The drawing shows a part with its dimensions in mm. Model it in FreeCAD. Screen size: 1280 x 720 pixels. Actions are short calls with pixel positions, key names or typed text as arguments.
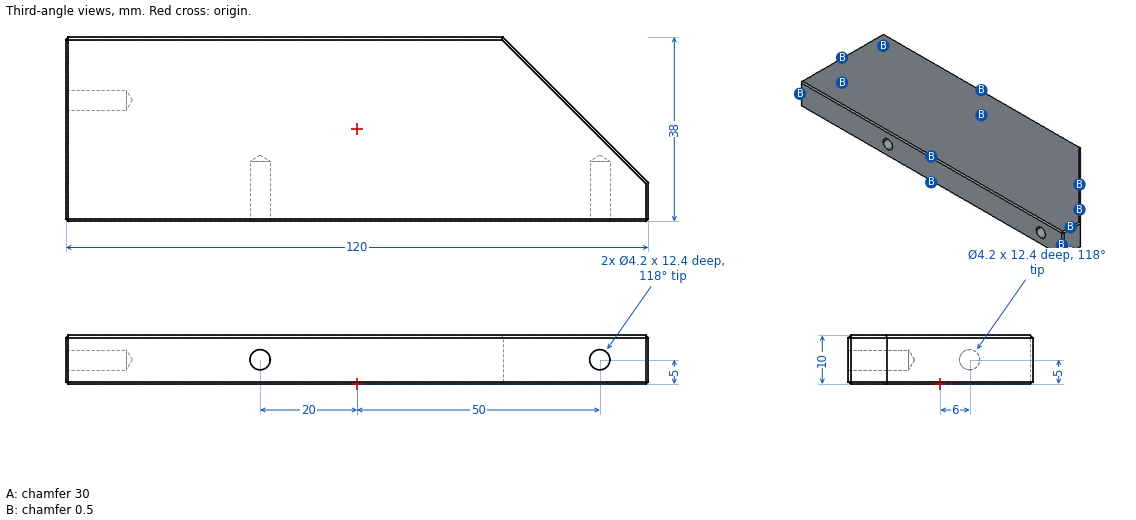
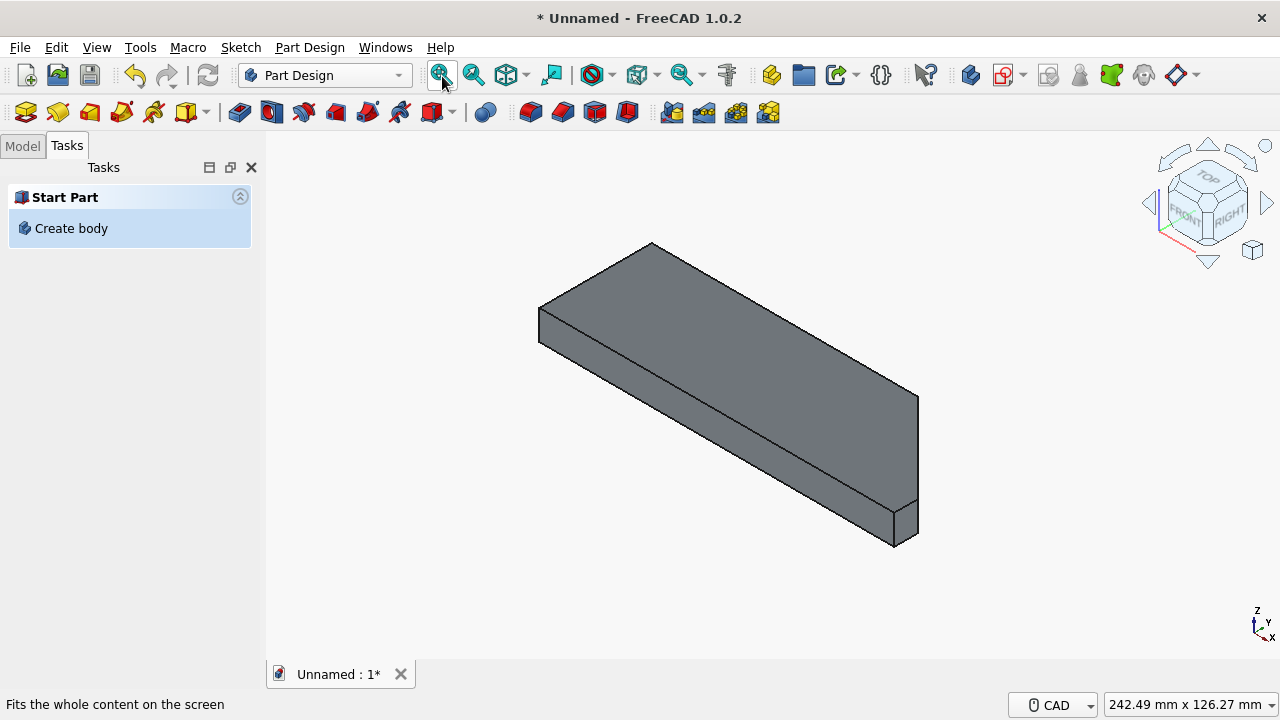
click(869, 514)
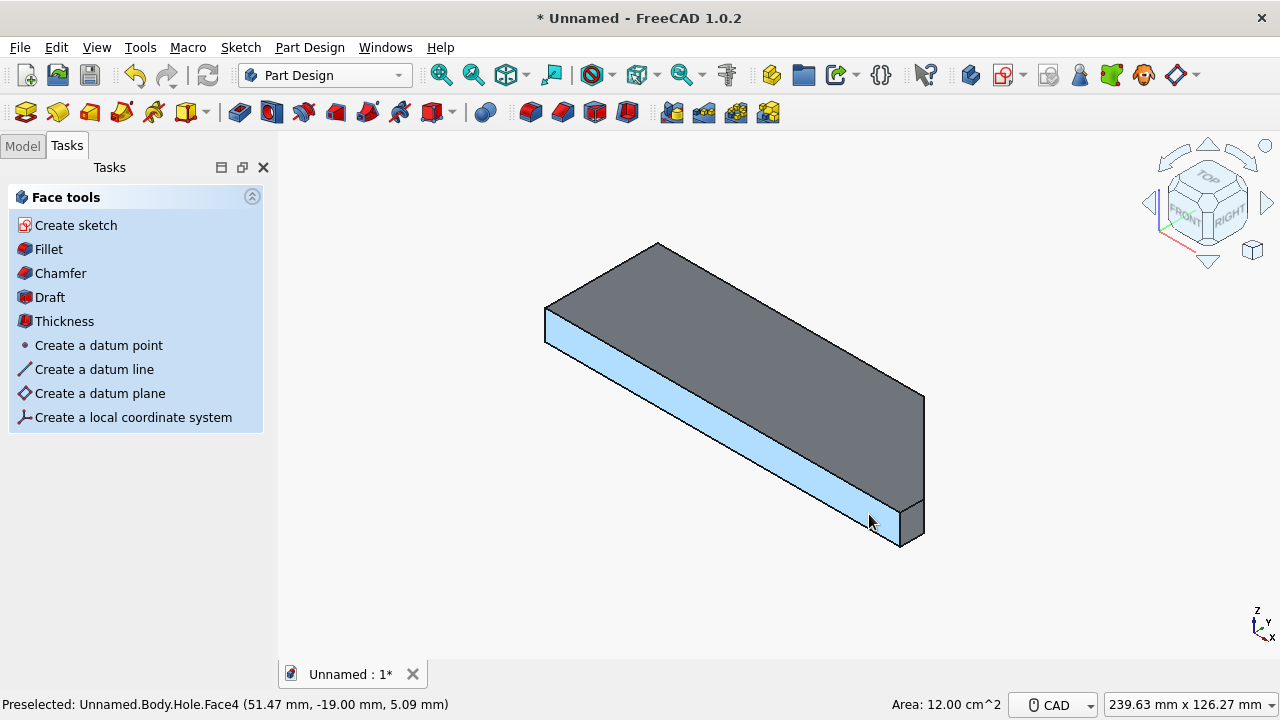
click(1004, 76)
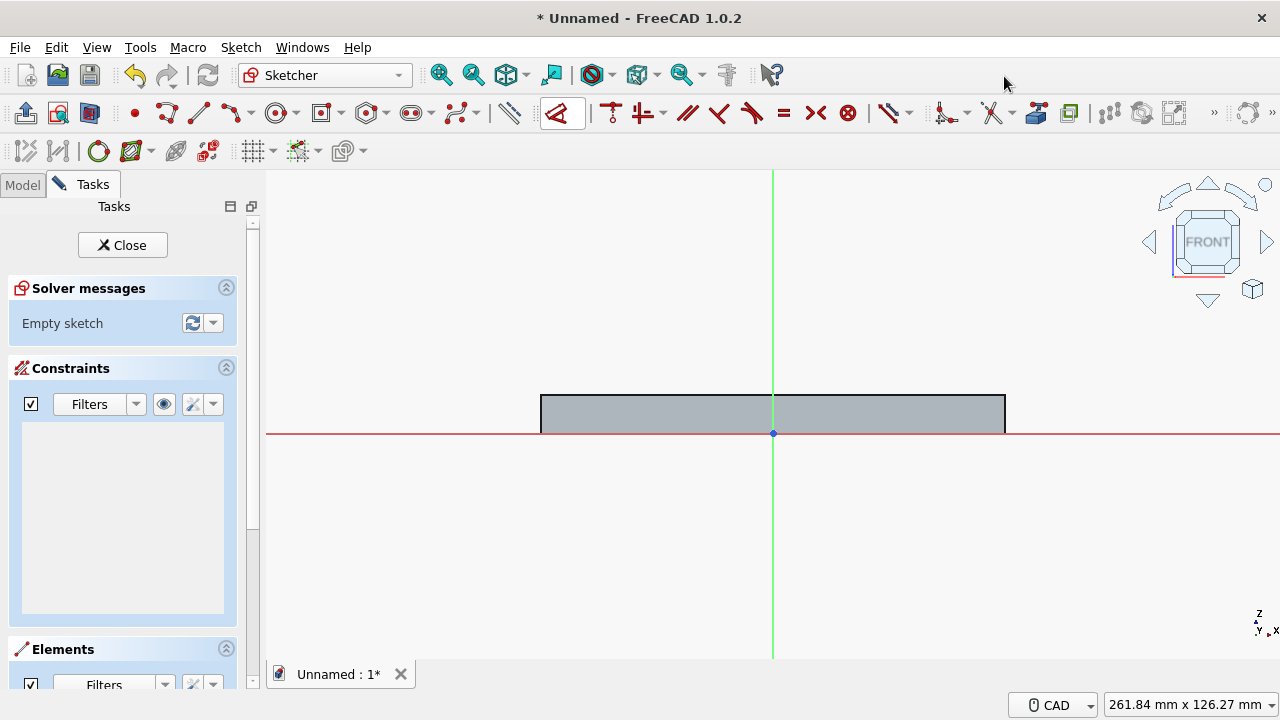
scroll(934, 425, up, 4)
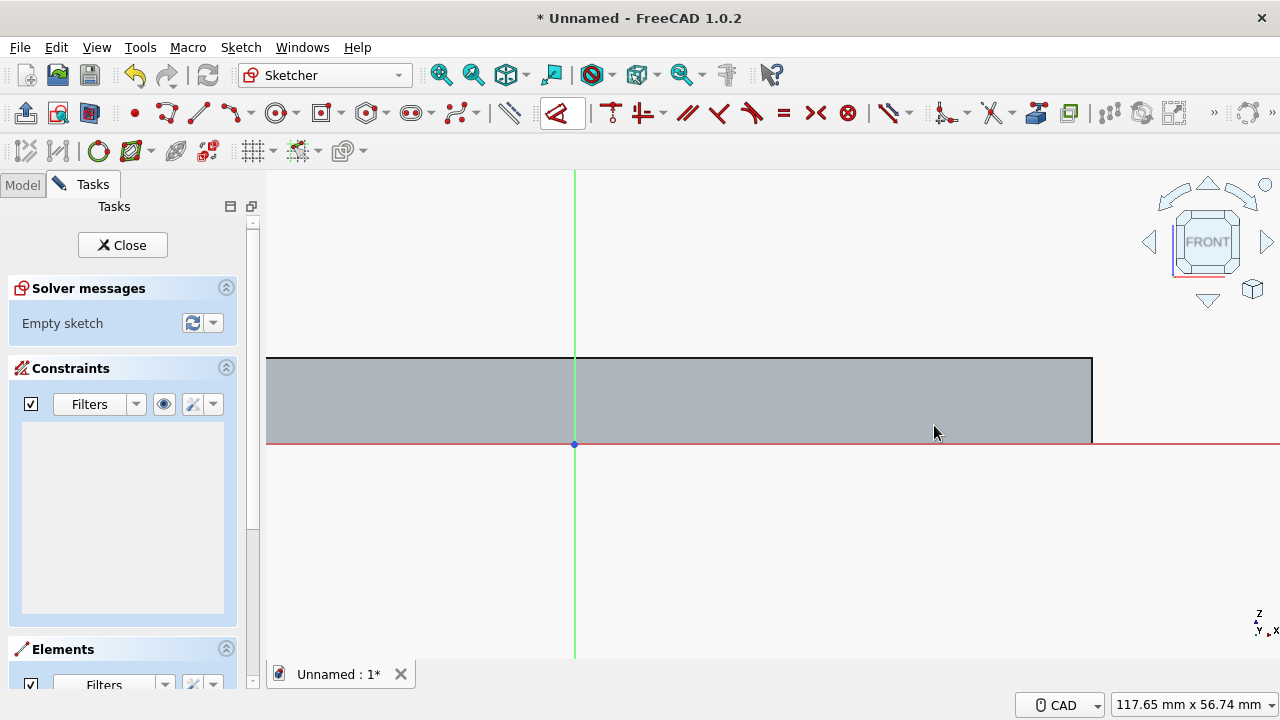
click(276, 114)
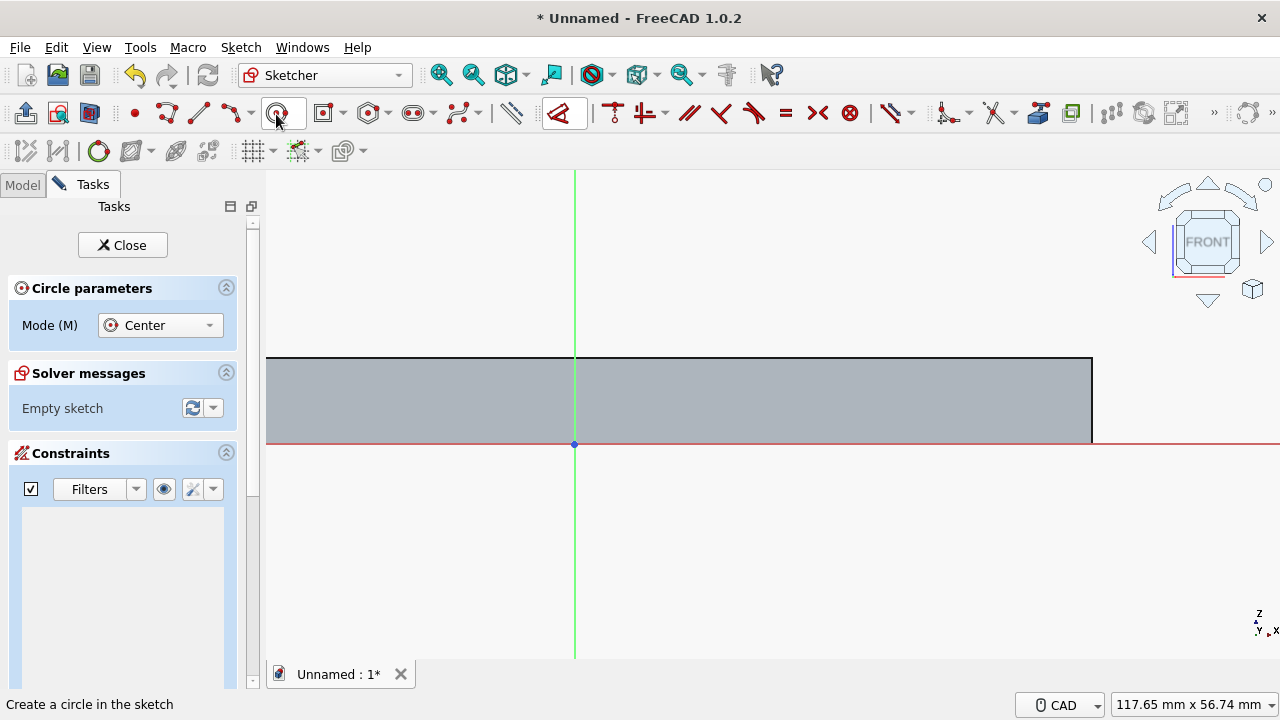
scroll(1006, 401, up, 2)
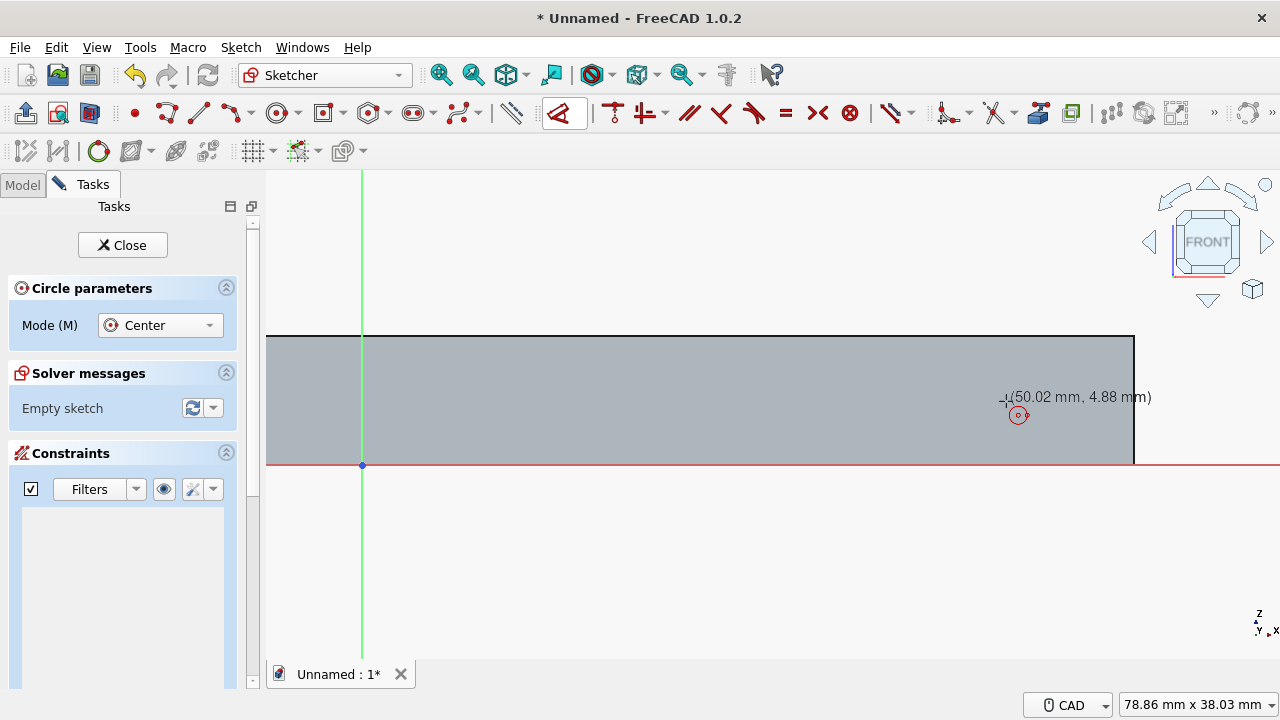
click(1005, 401)
click(1024, 382)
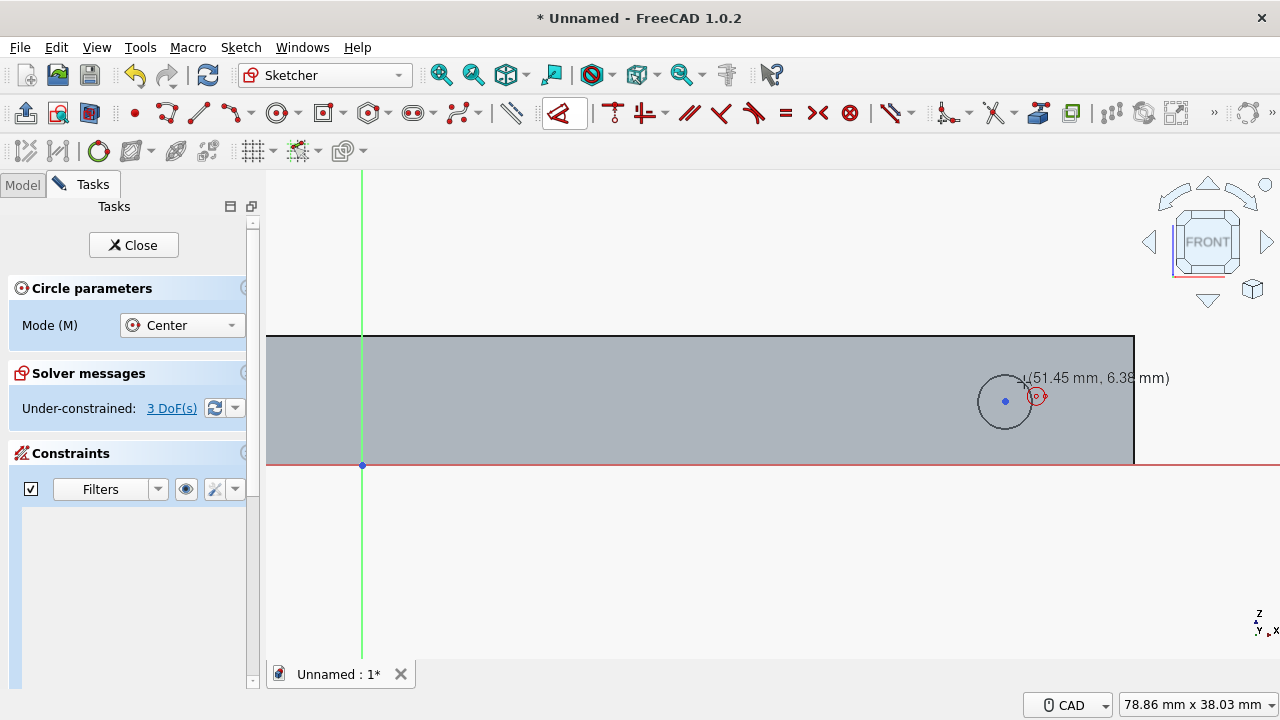
scroll(1008, 405, down, 2)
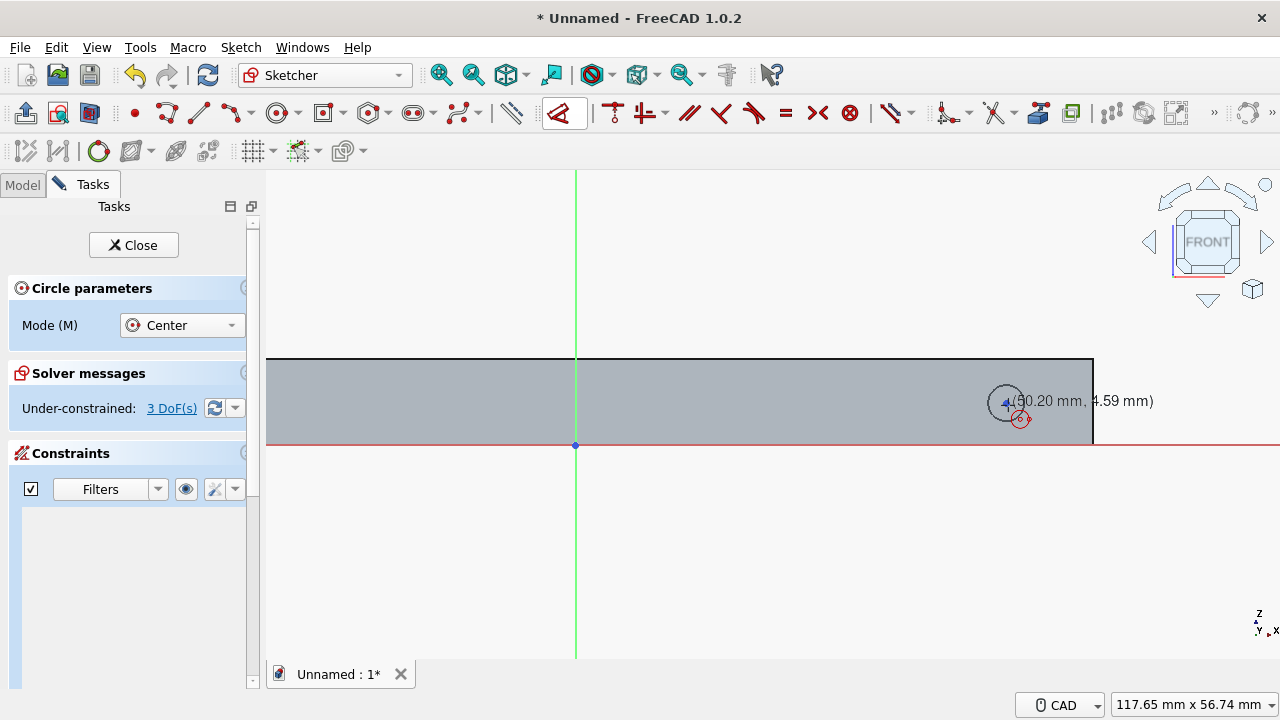
scroll(403, 402, up, 2)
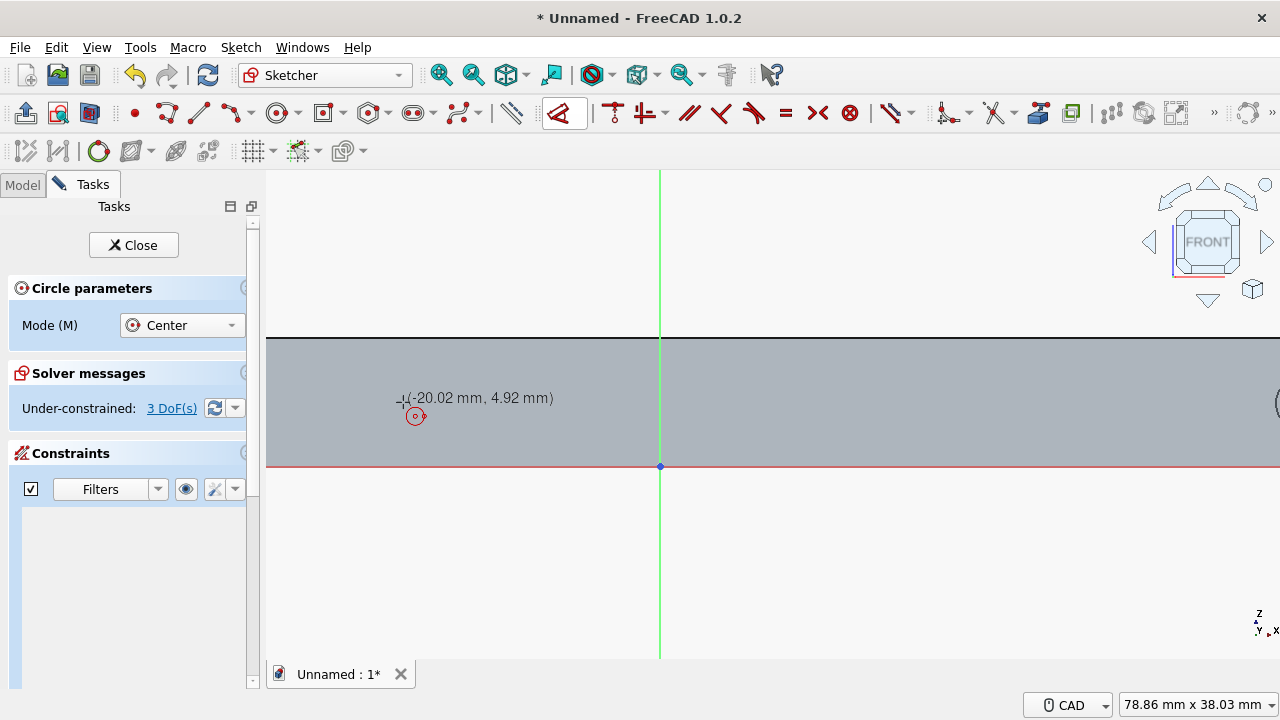
click(403, 402)
click(422, 383)
key(Escape)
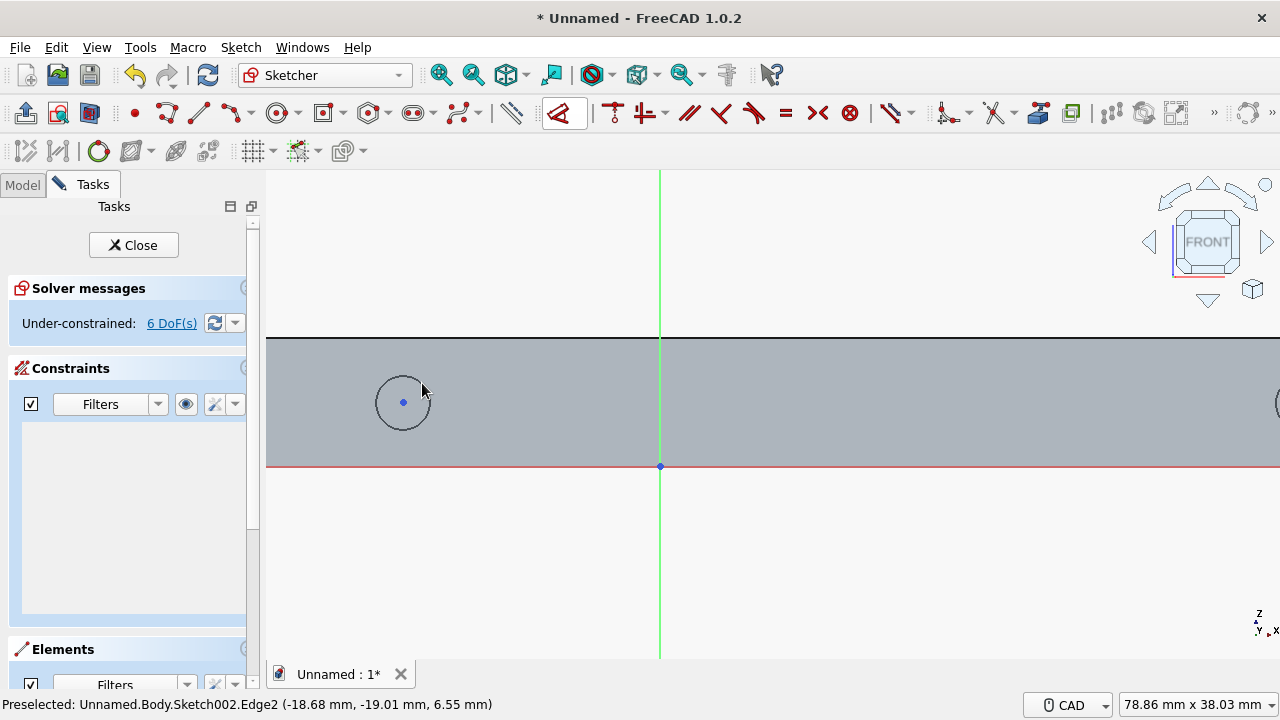
scroll(402, 402, down, 2)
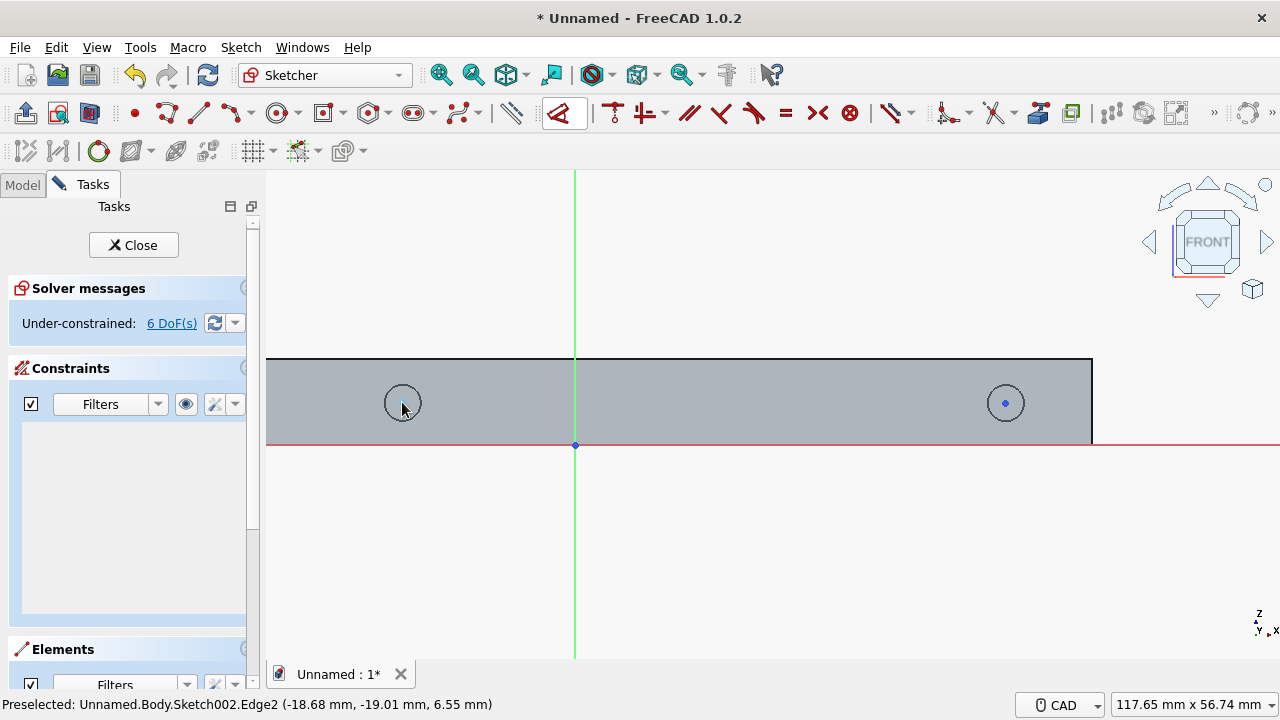
click(1019, 390)